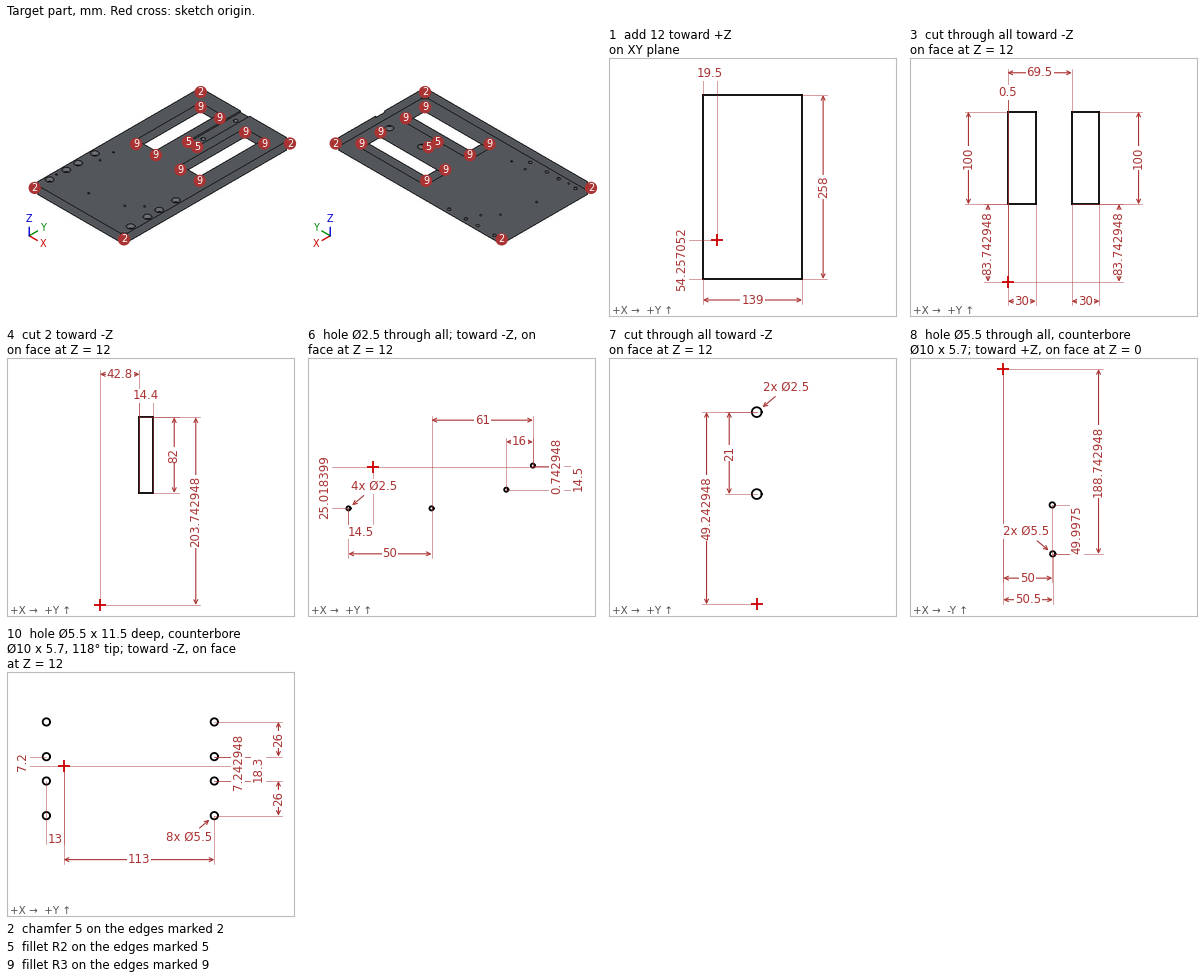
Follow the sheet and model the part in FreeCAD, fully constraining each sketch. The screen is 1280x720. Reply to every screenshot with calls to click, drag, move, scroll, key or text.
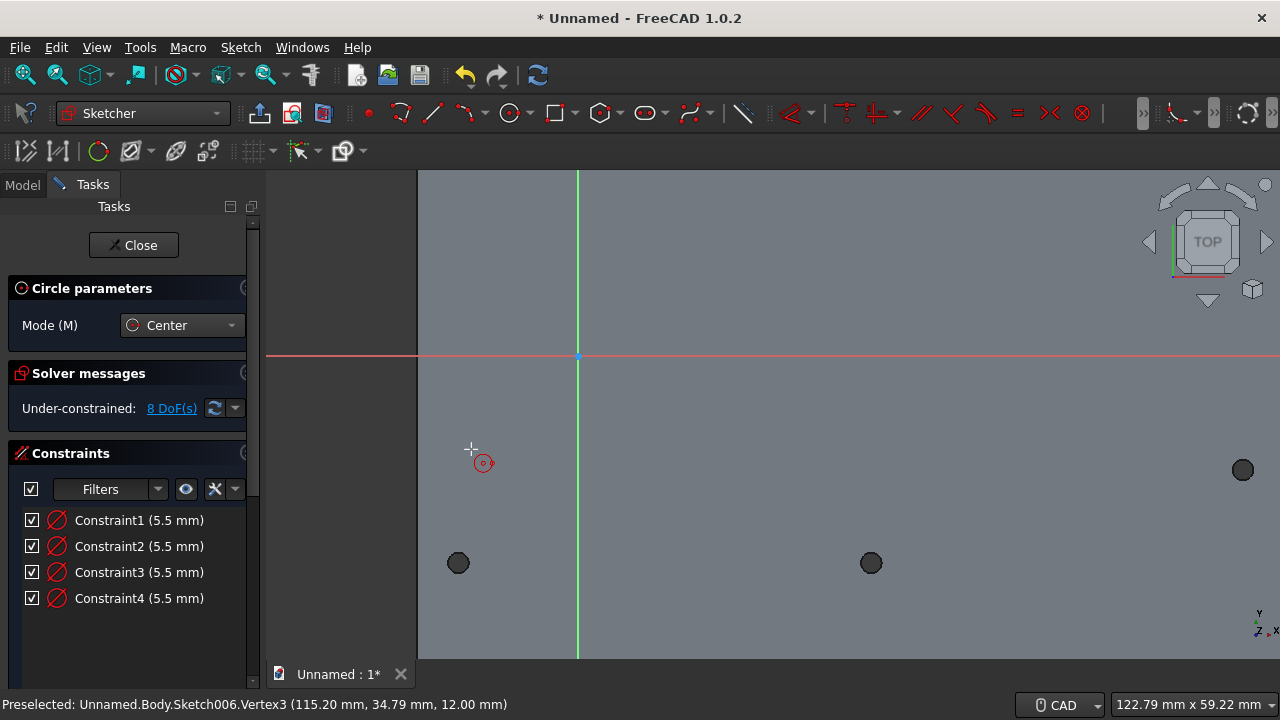
click(471, 448)
move(487, 432)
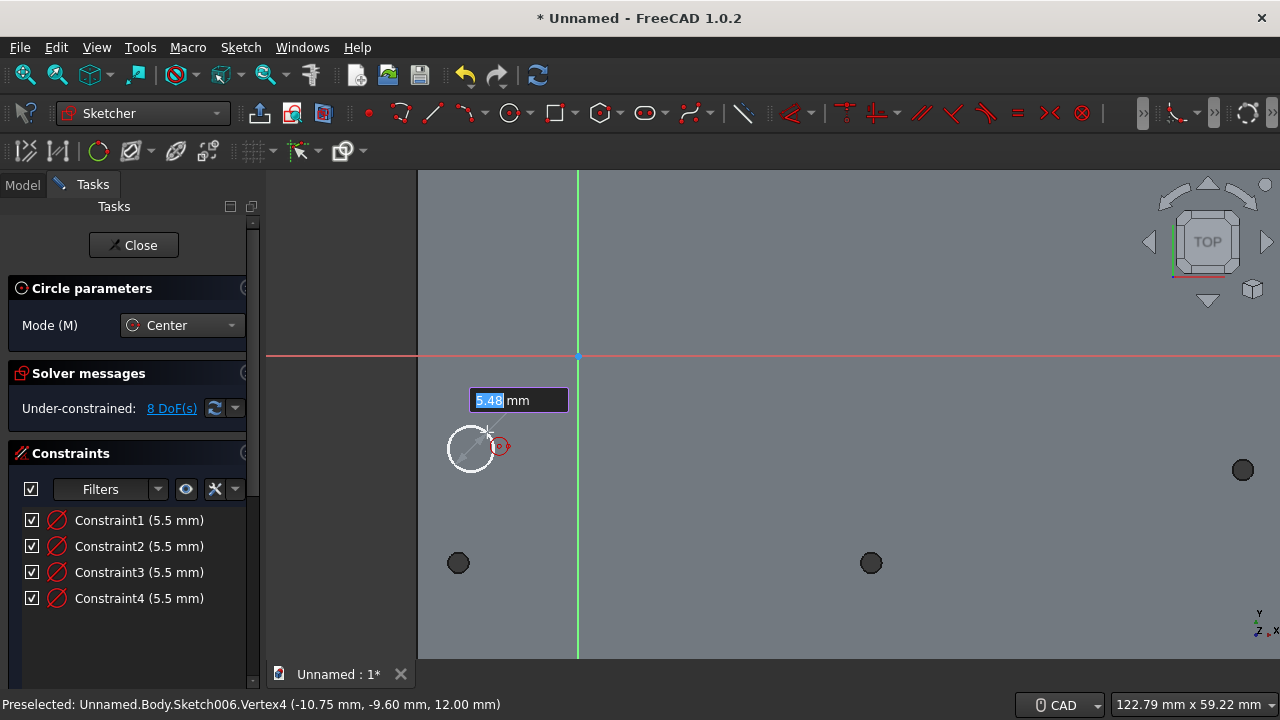
text(5.5)
key(Return)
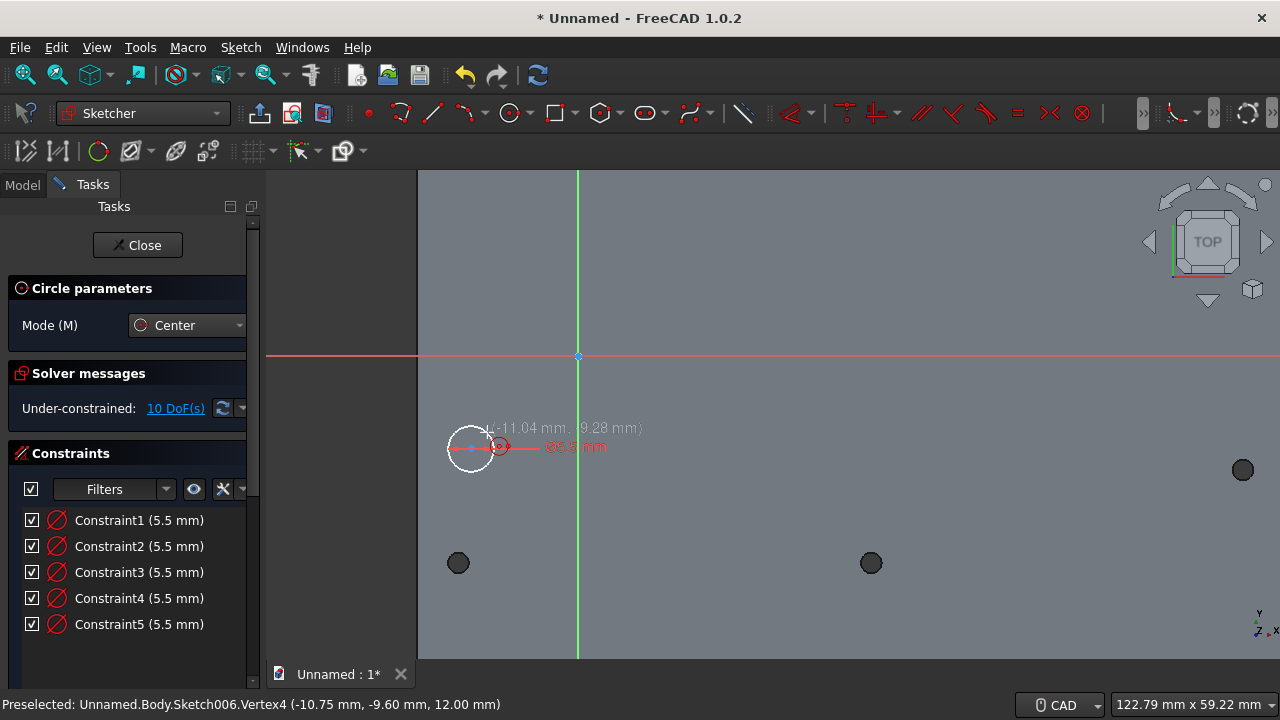
click(471, 297)
move(487, 281)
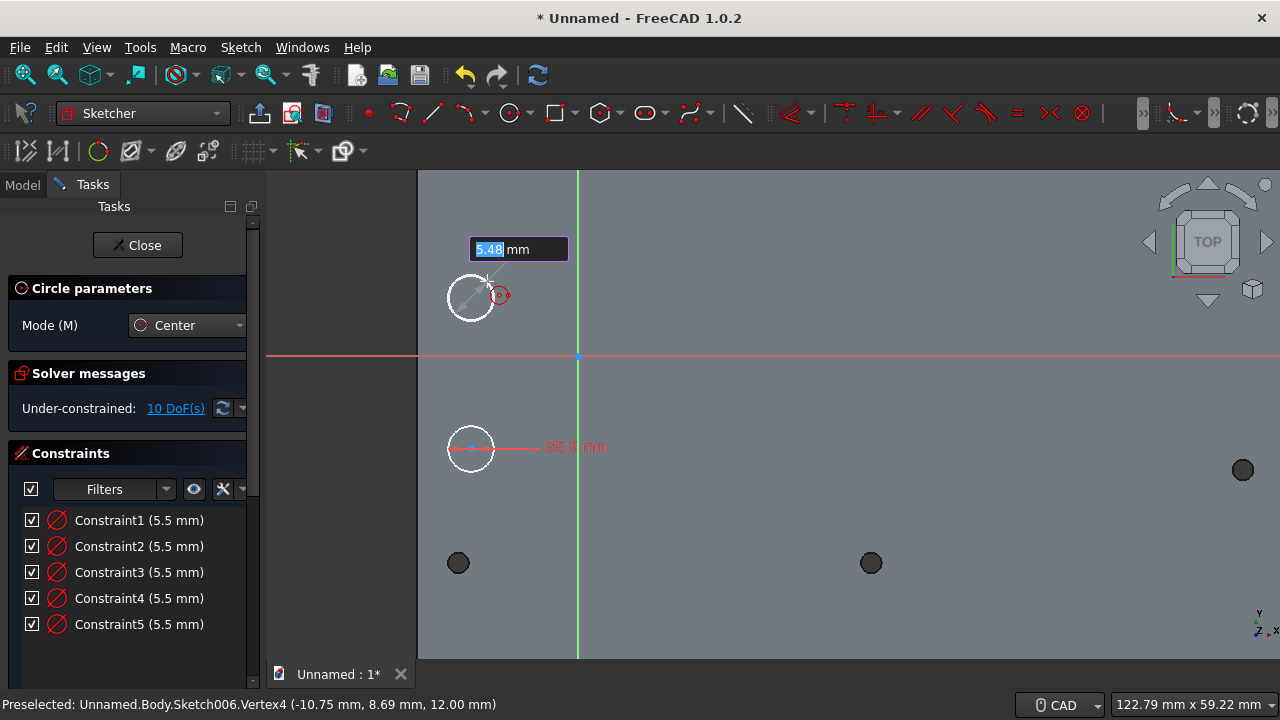
text(5.5)
key(Return)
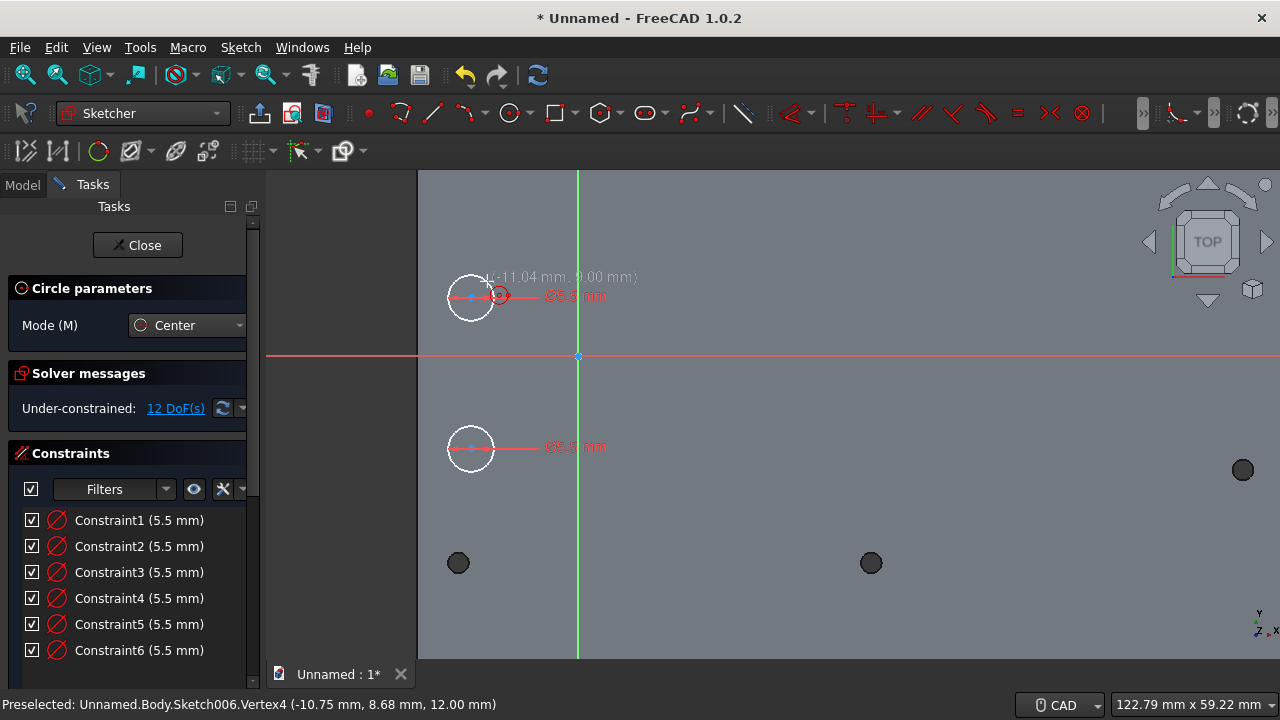
scroll(471, 449, down, 4)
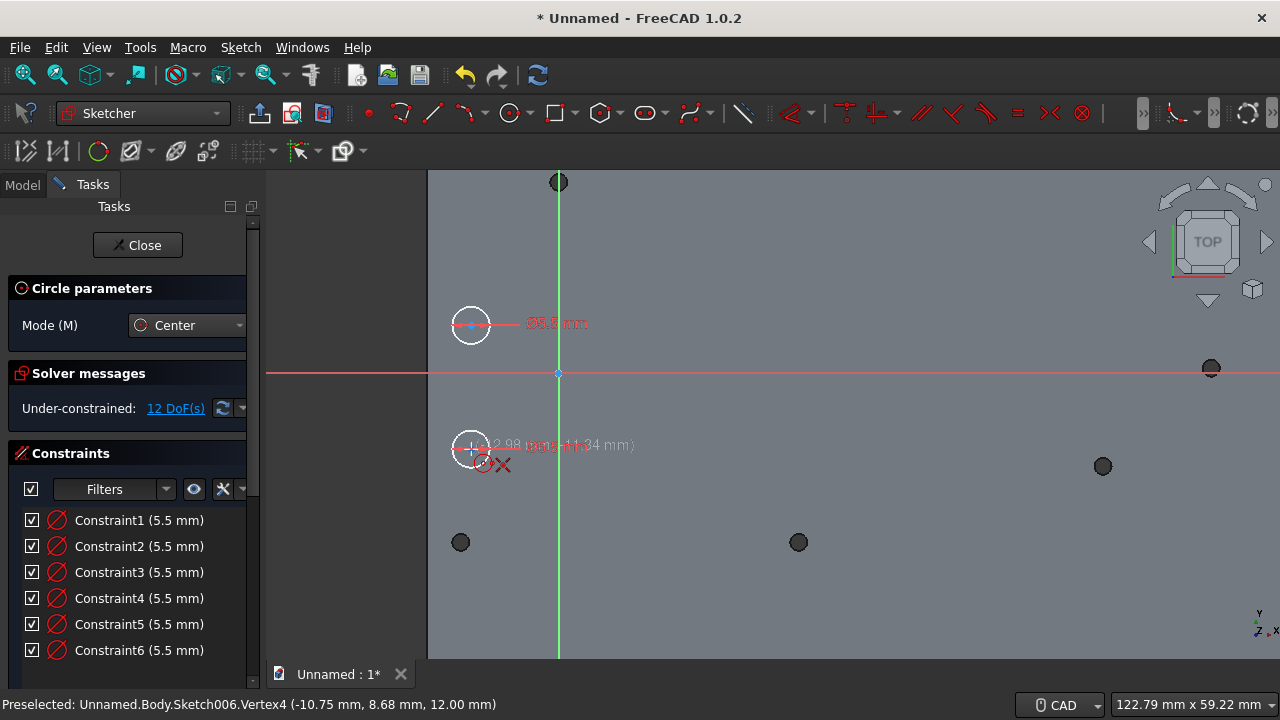
scroll(471, 545, up, 4)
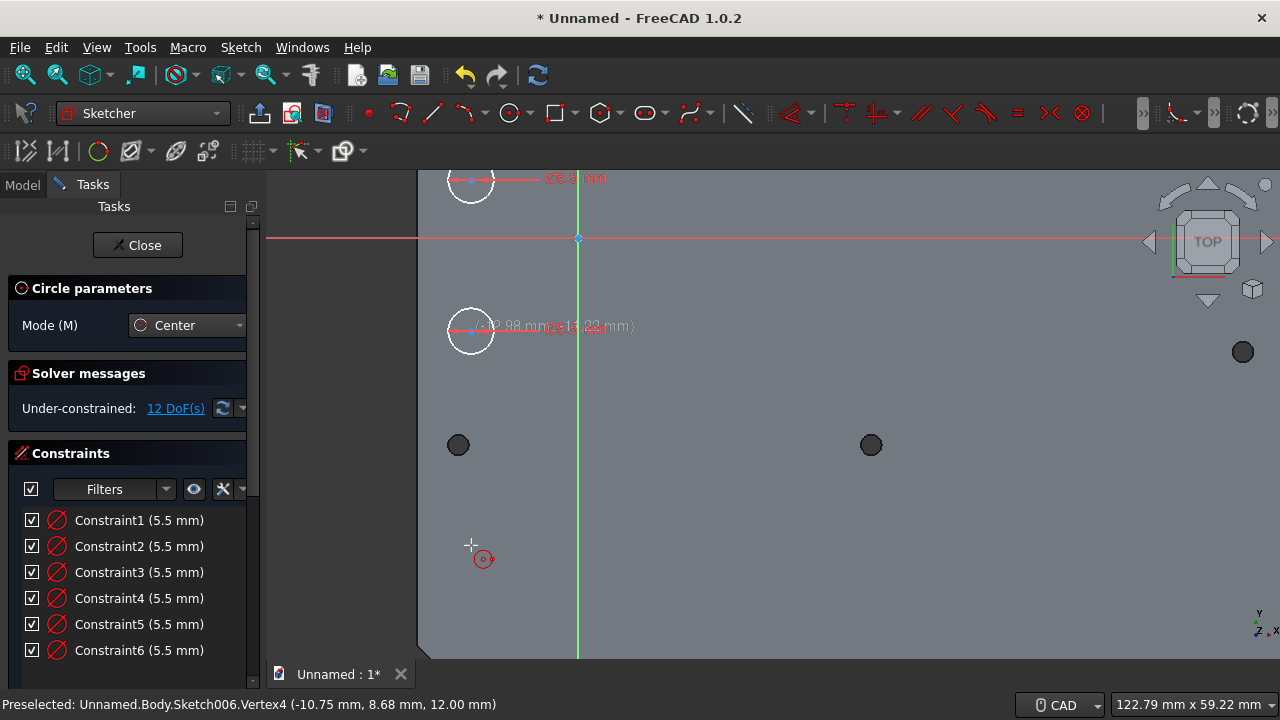
click(471, 544)
move(487, 528)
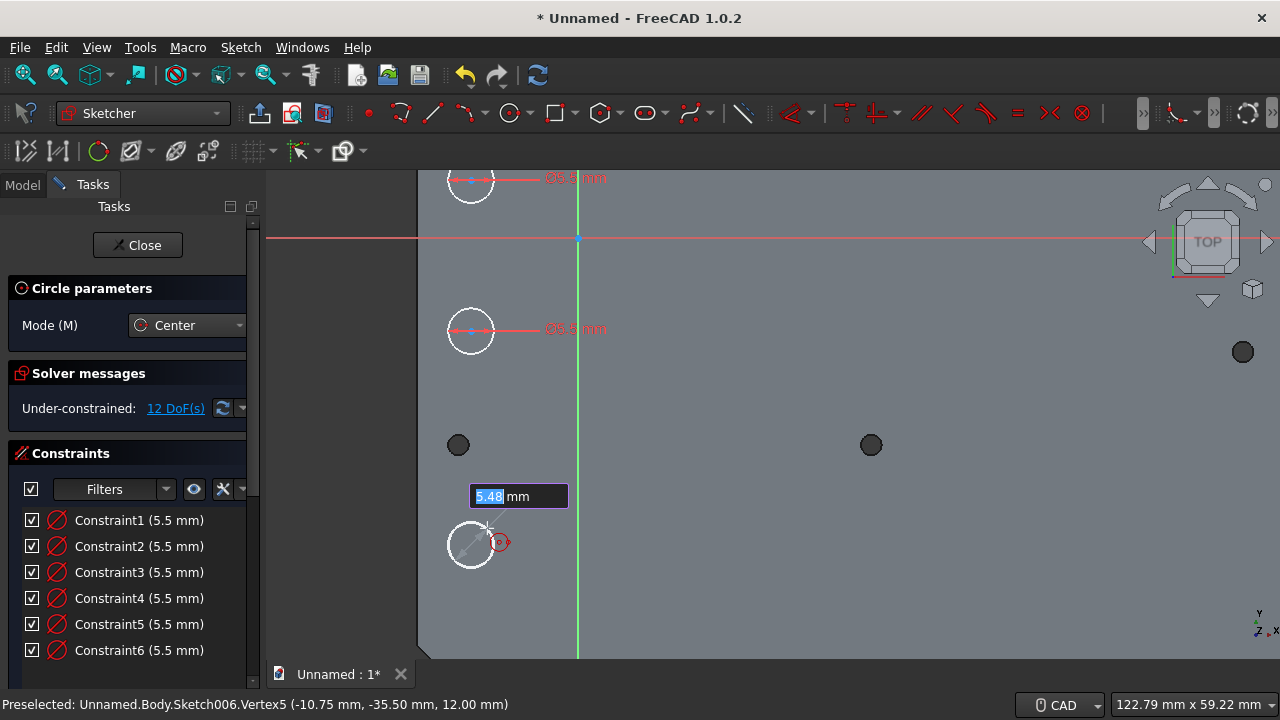
text(5.5)
key(Return)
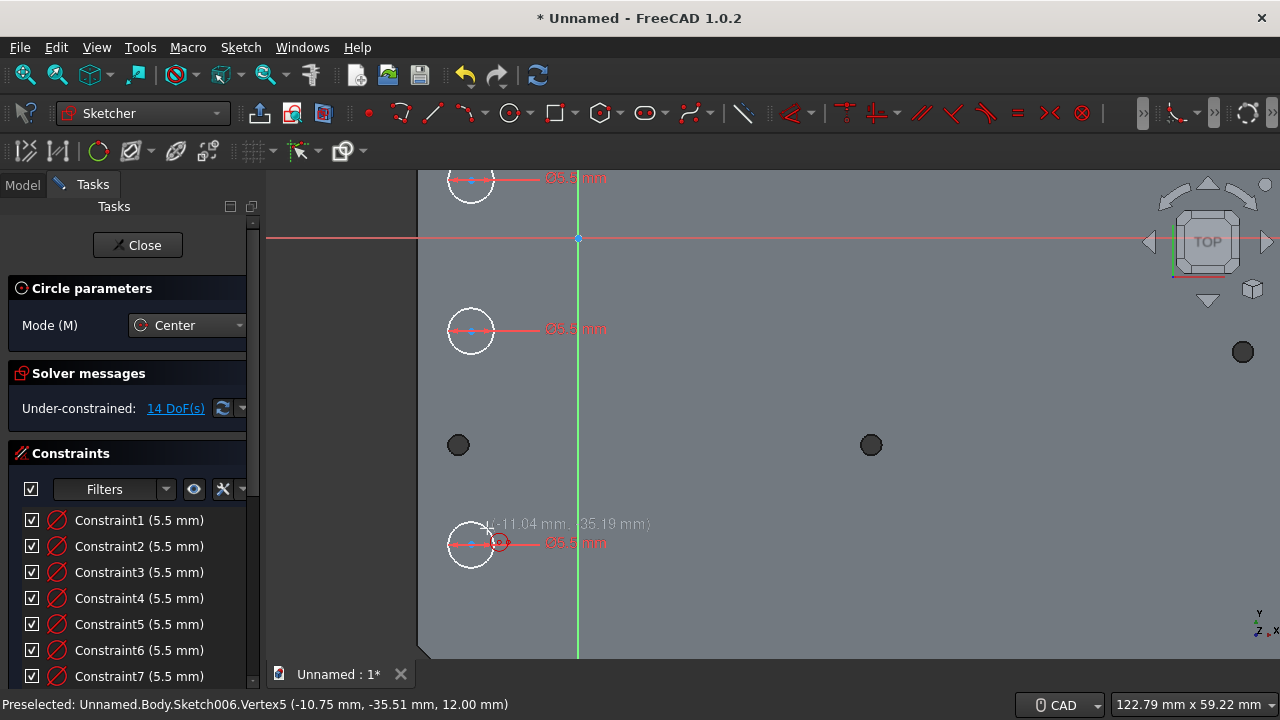
scroll(471, 545, down, 4)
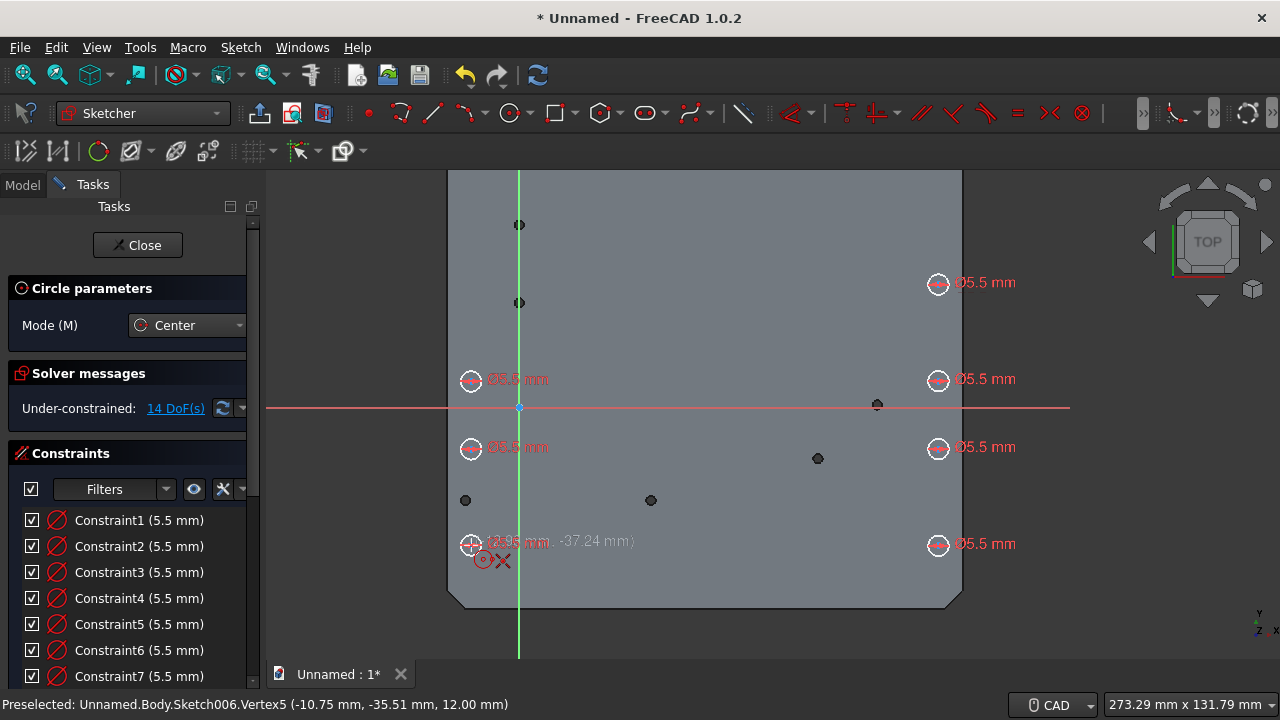
scroll(471, 284, up, 4)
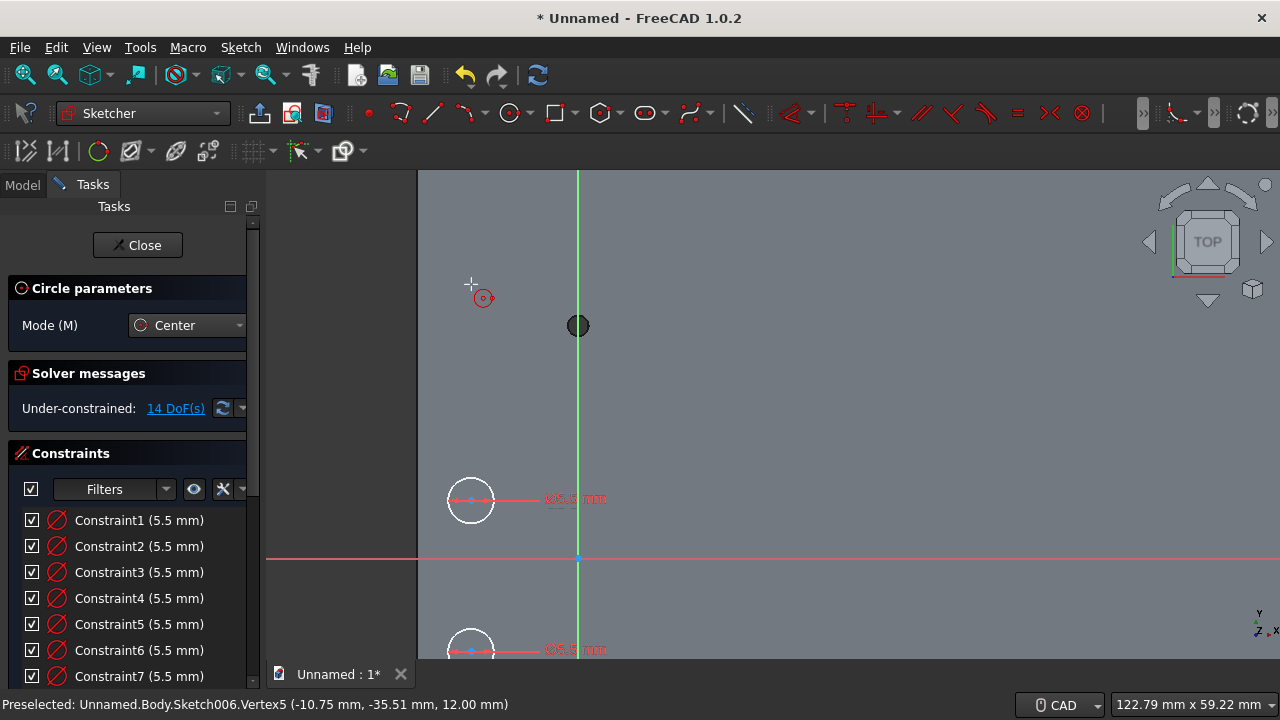
click(471, 284)
move(487, 268)